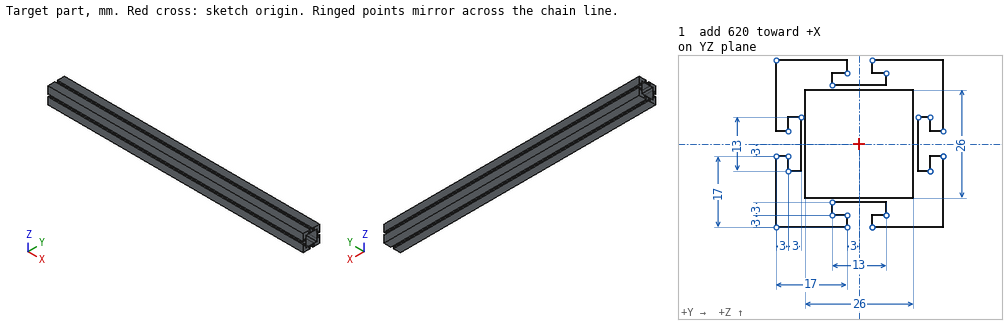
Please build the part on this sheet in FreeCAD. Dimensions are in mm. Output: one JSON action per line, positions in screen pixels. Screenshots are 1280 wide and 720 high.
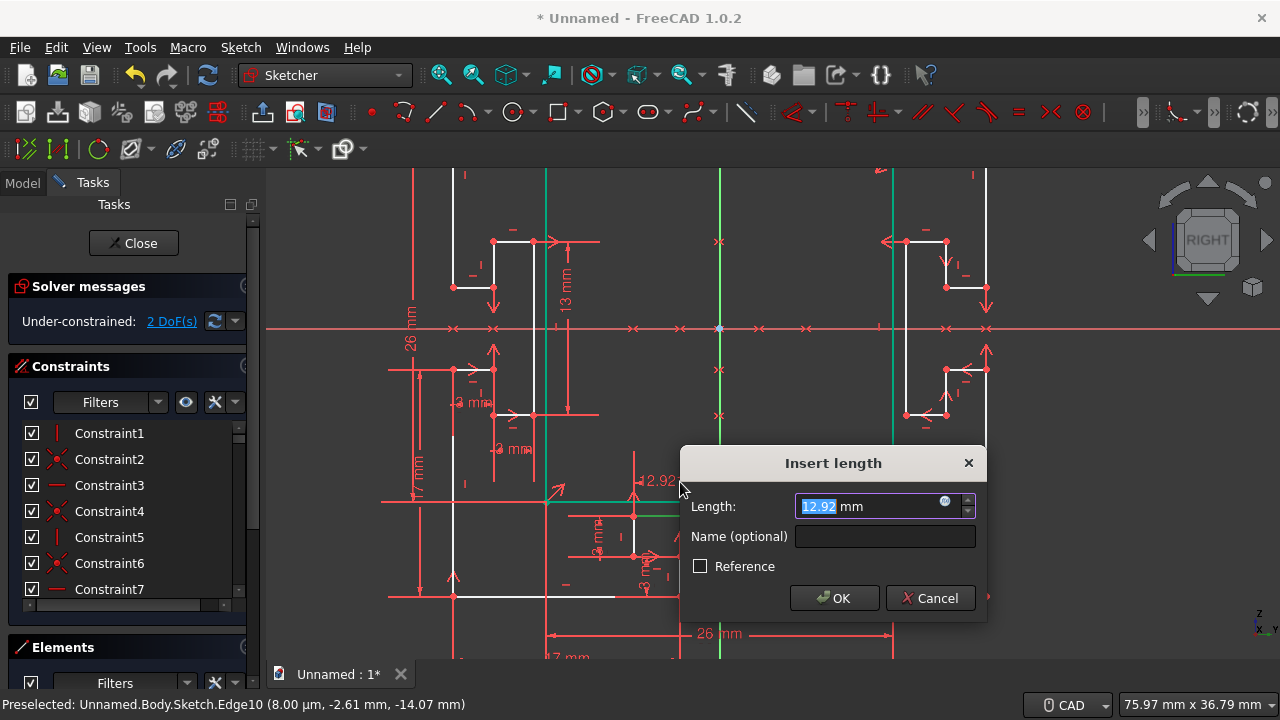
{"action": "type", "text": "13"}
{"action": "key", "text": "Return"}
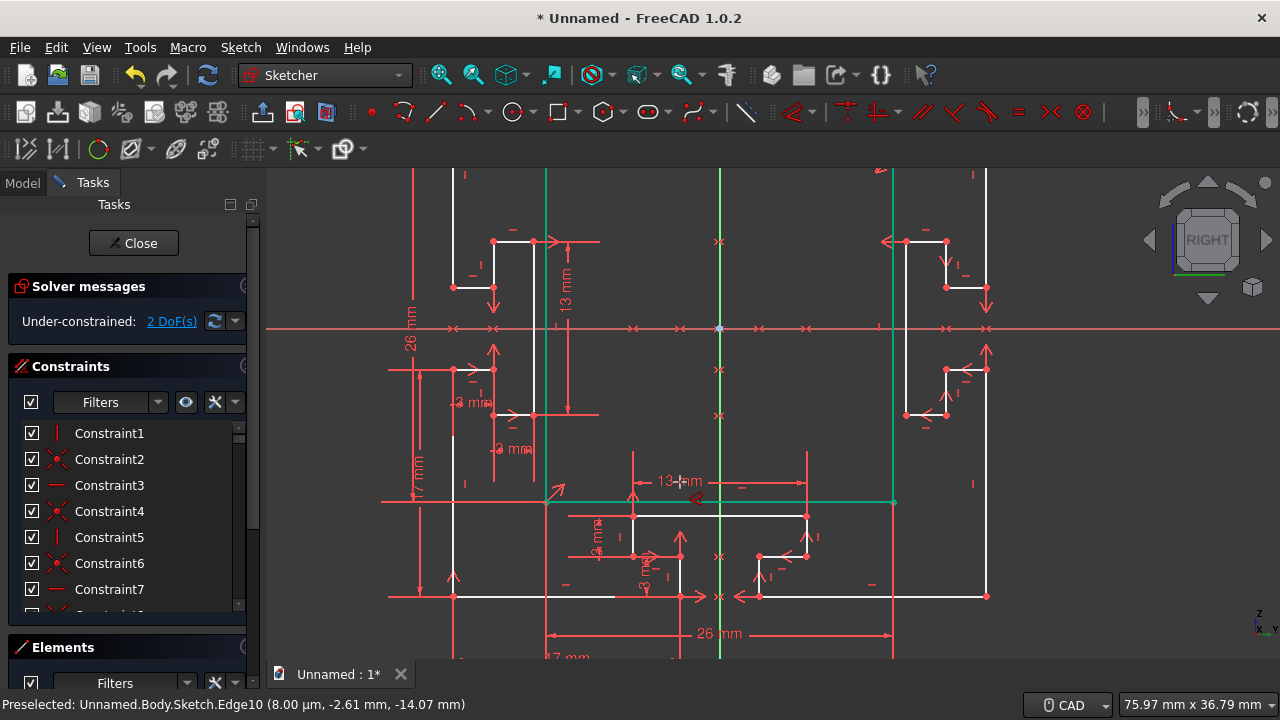
{"action": "left_click", "coordinate": [494, 370]}
{"action": "left_click", "coordinate": [460, 349]}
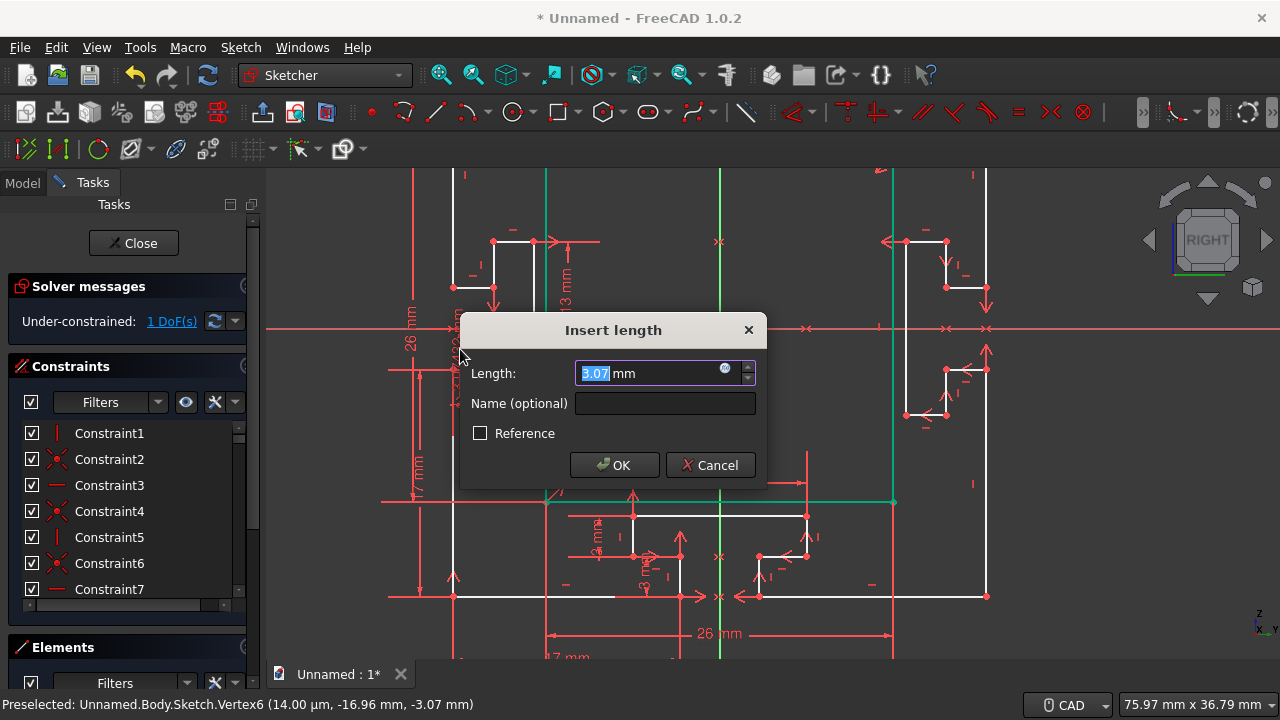
{"action": "type", "text": "3"}
{"action": "key", "text": "Return"}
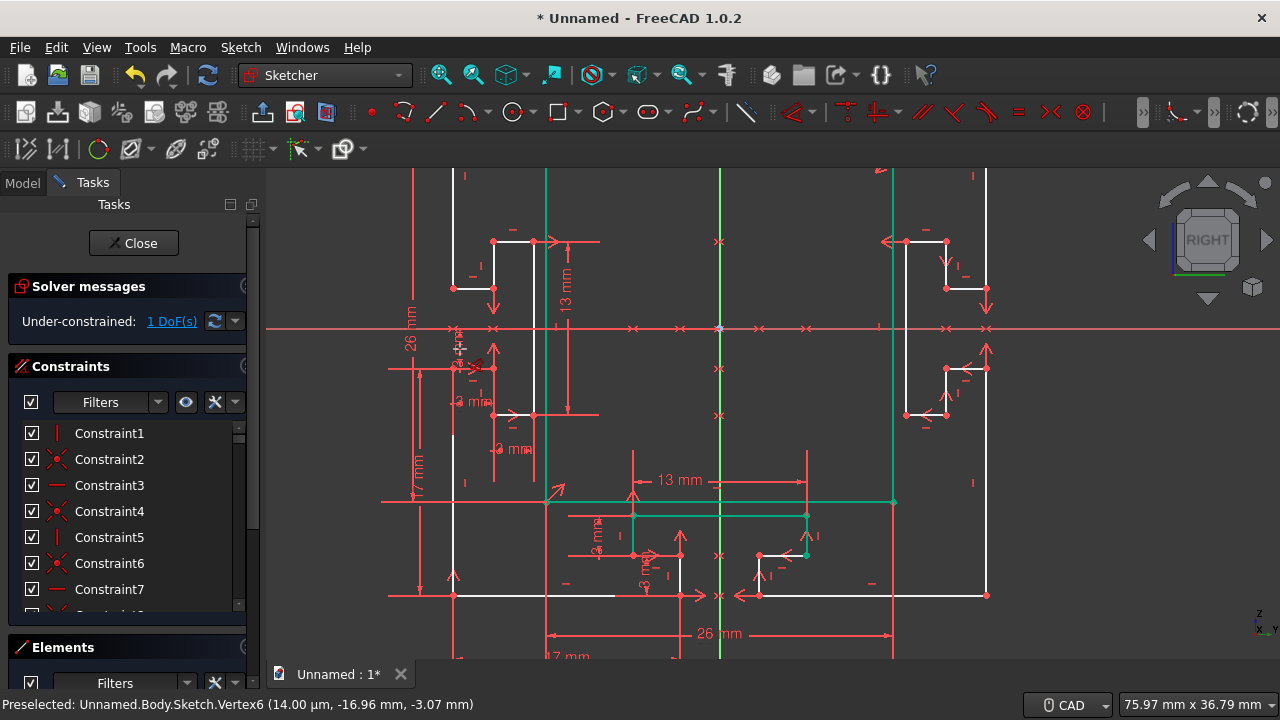
{"action": "left_click", "coordinate": [680, 596]}
{"action": "left_click", "coordinate": [700, 630]}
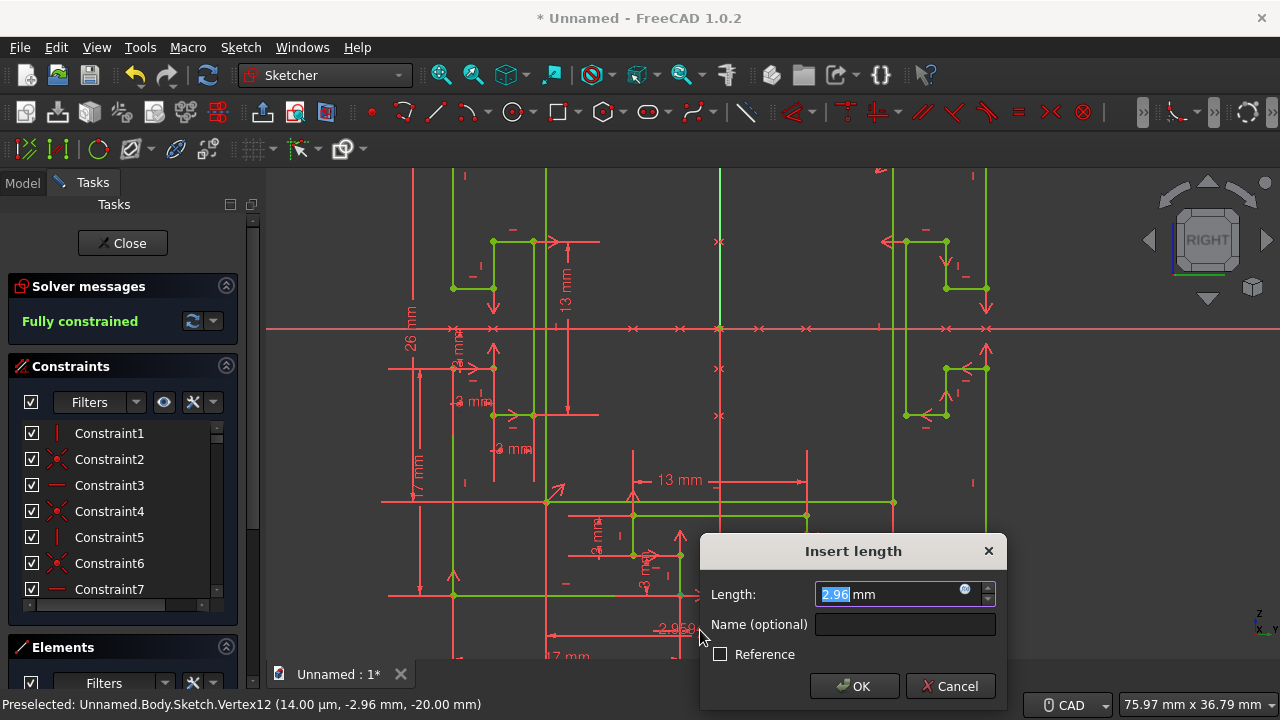
{"action": "type", "text": "3"}
{"action": "key", "text": "Return"}
{"action": "key", "text": "Escape"}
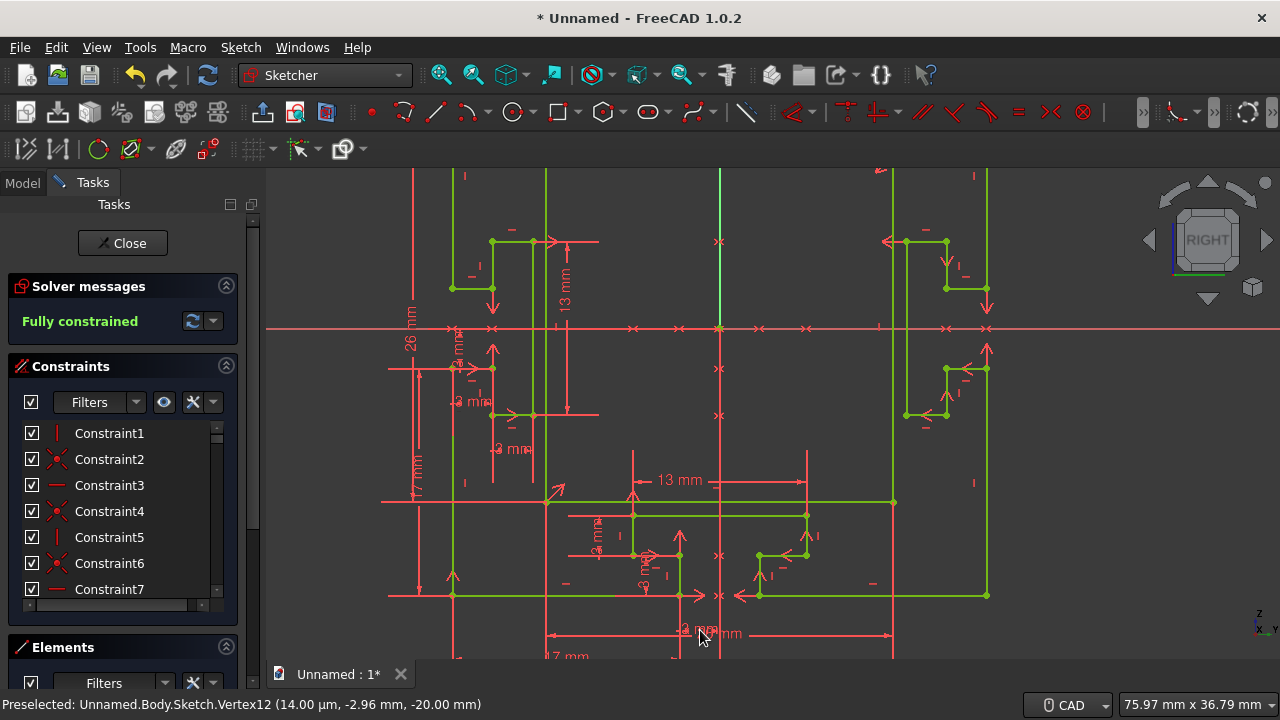
{"action": "left_click", "coordinate": [123, 243]}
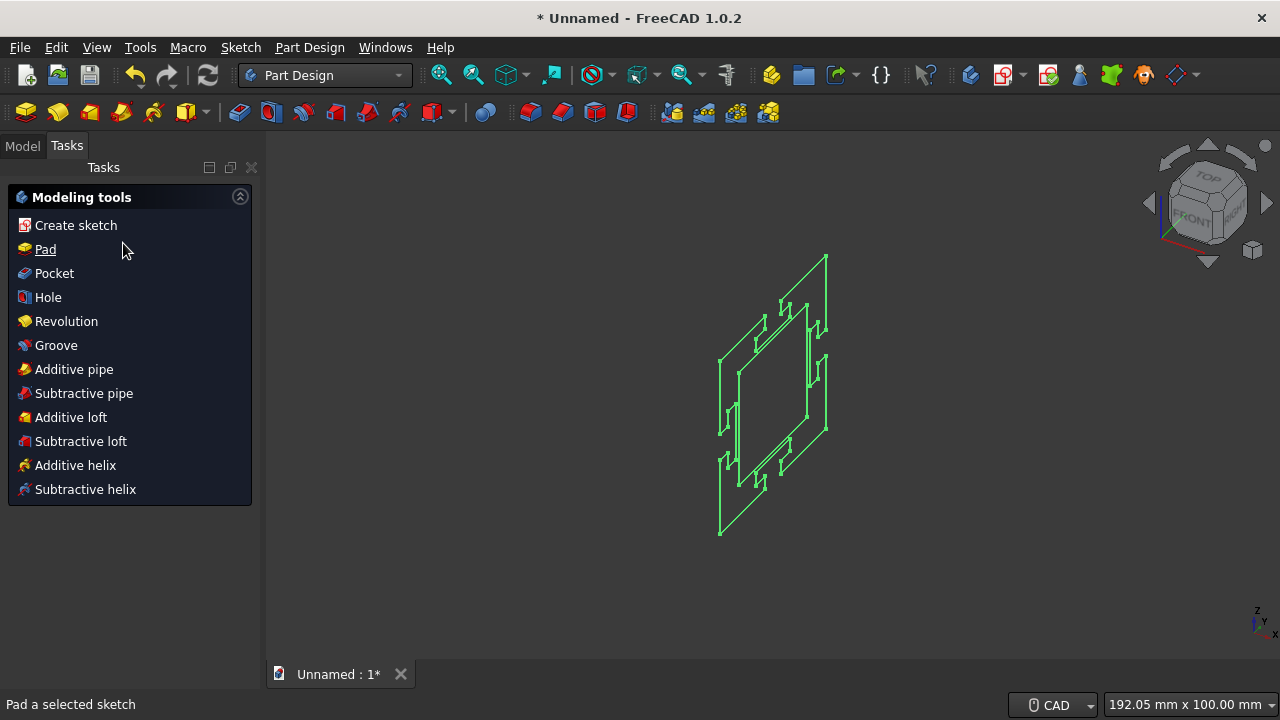
{"action": "left_click", "coordinate": [26, 112]}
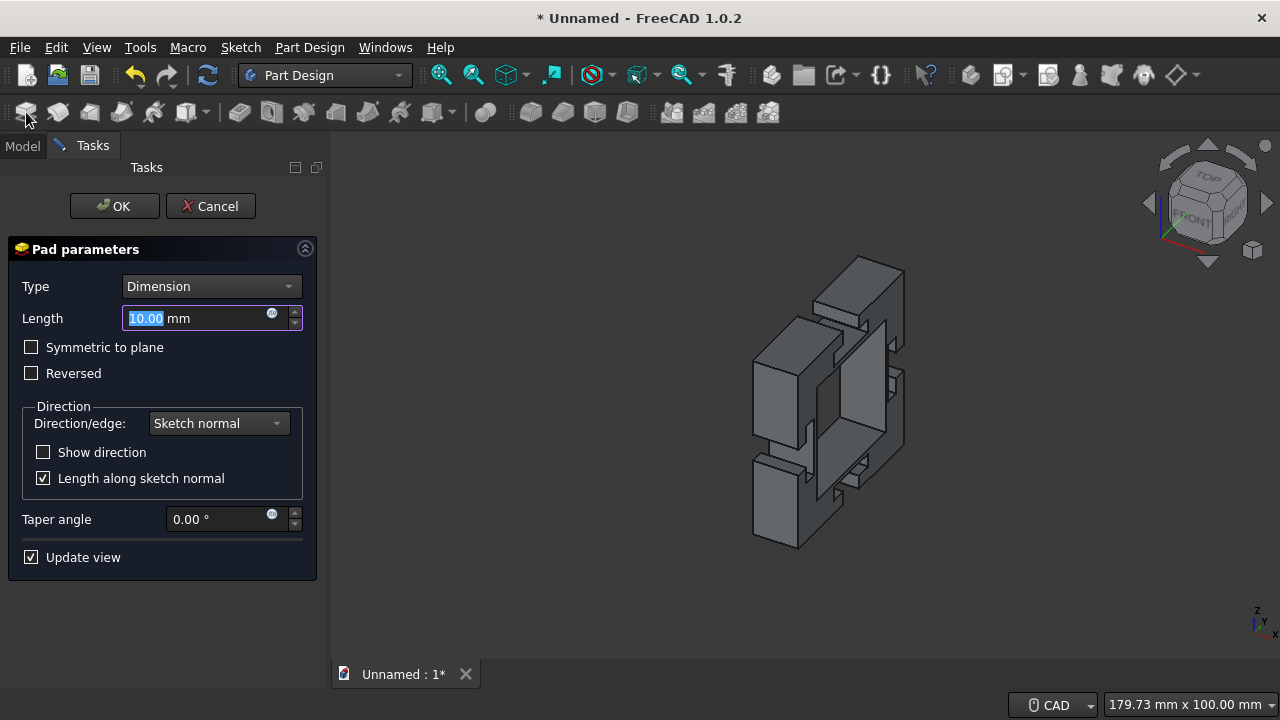
{"action": "type", "text": "620"}
{"action": "key", "text": "Tab"}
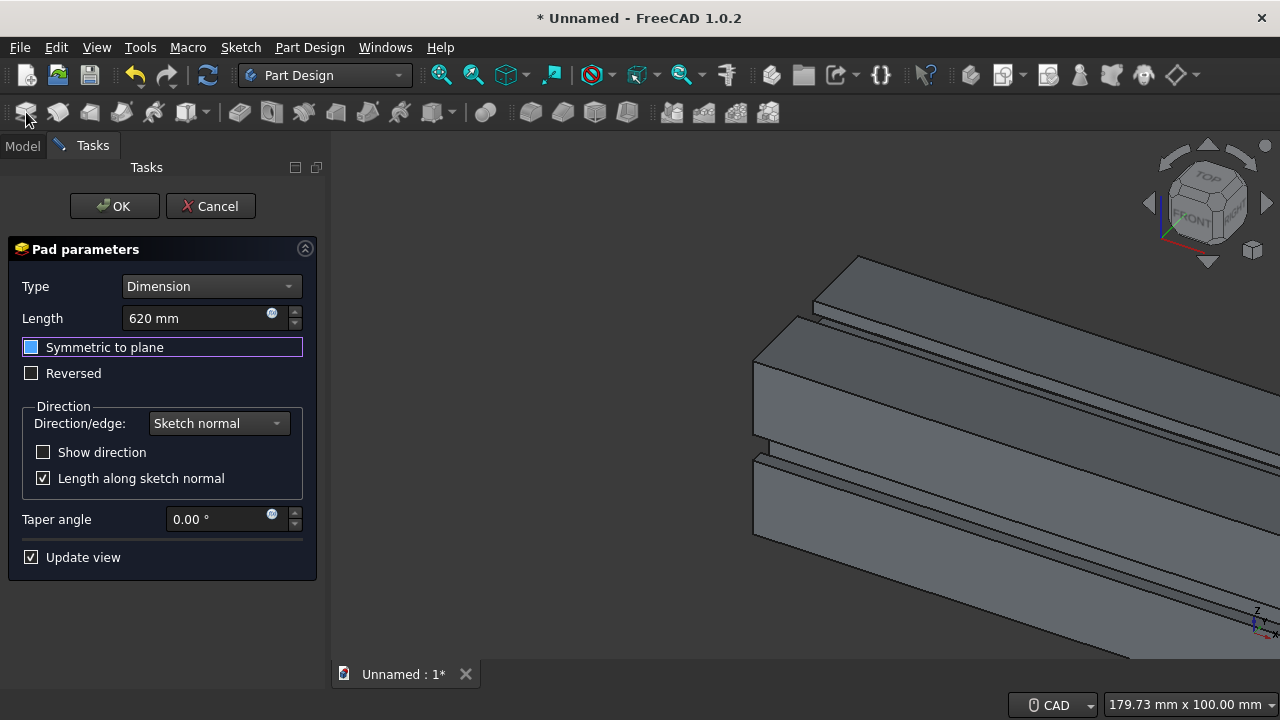
{"action": "left_click", "coordinate": [115, 206]}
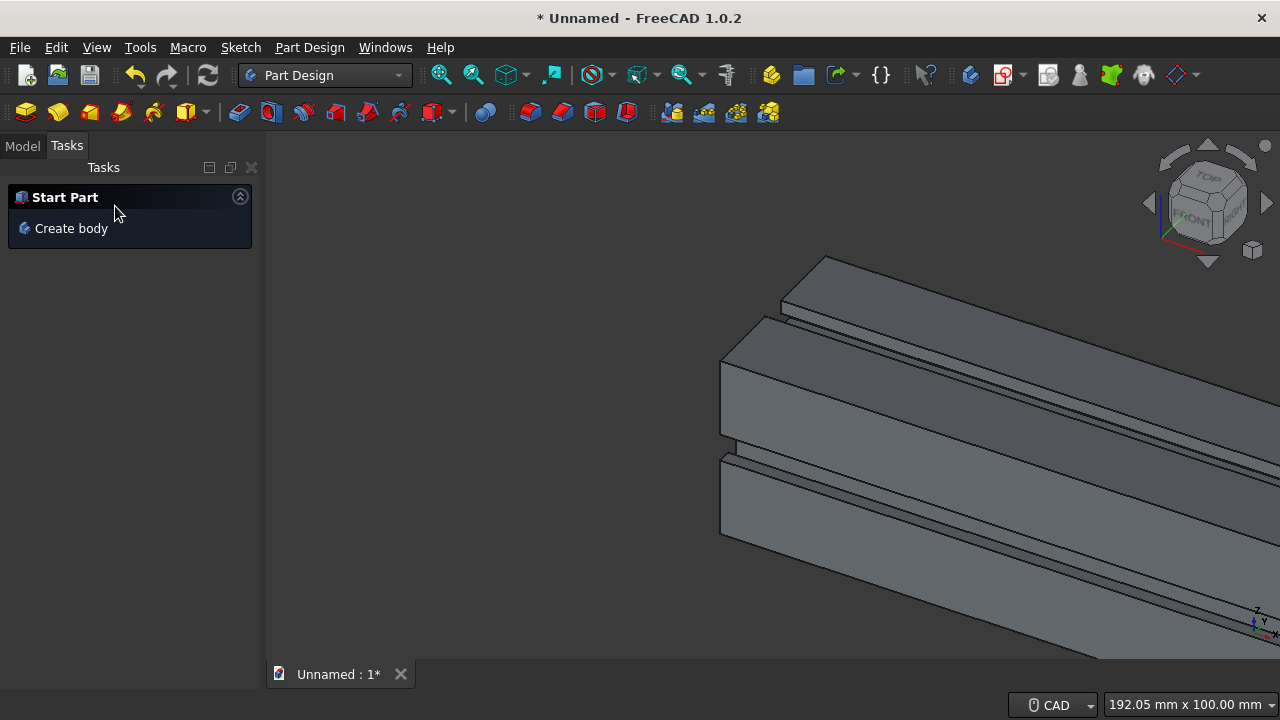
{"action": "key", "text": "0"}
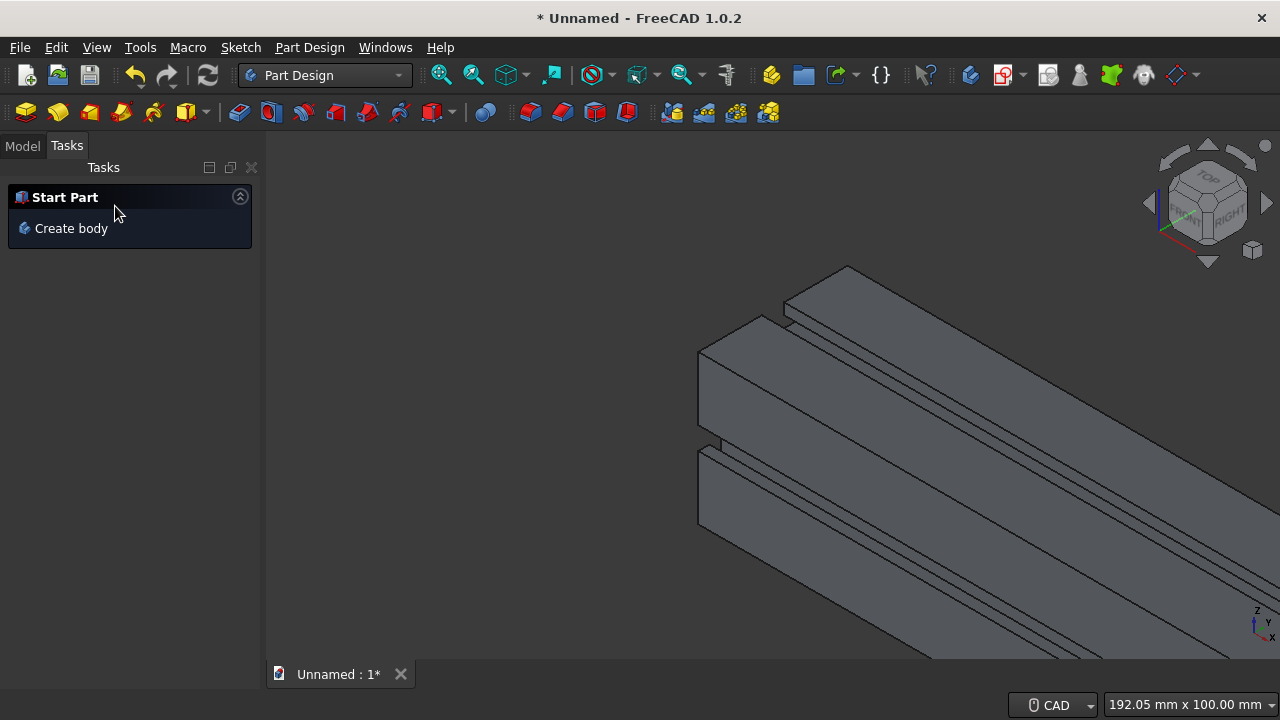
{"action": "key", "text": "v f"}